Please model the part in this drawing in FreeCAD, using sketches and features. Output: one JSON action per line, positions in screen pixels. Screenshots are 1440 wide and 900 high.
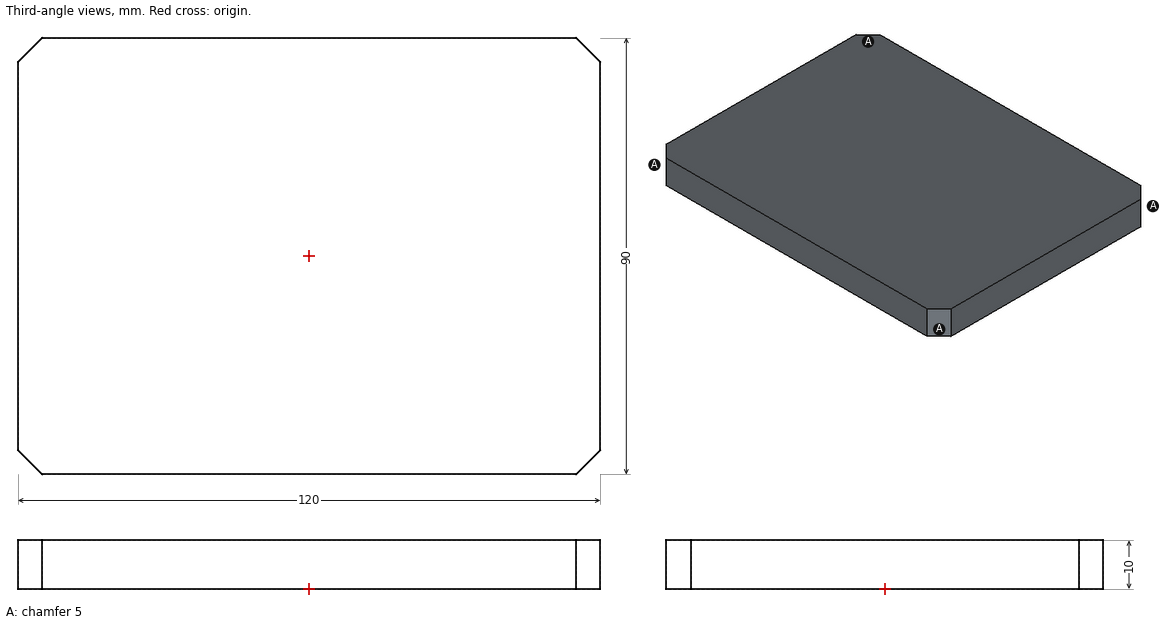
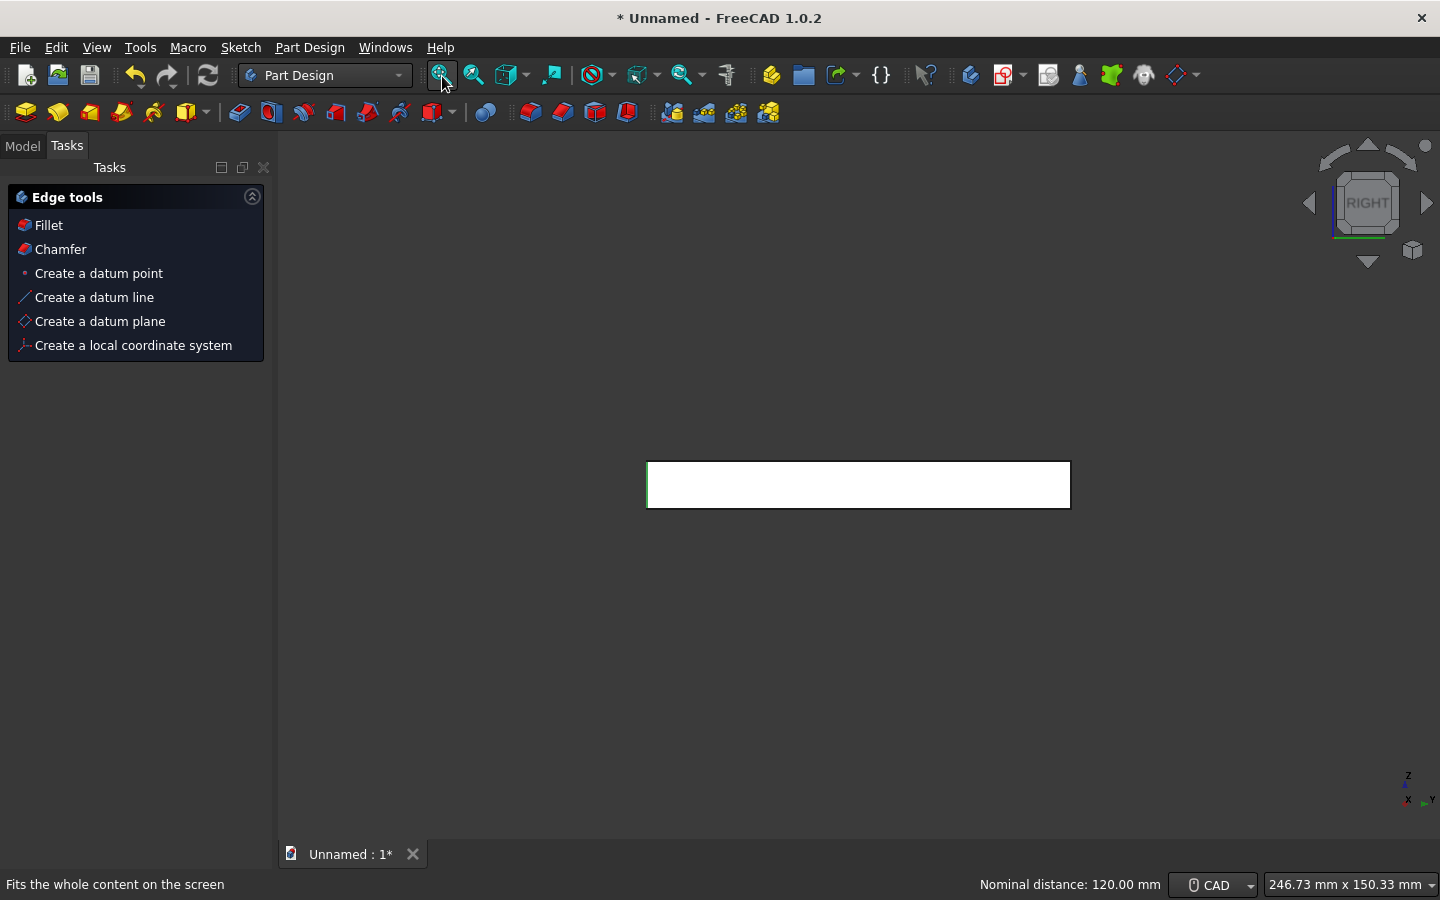
{"action": "left_click", "coordinate": [1071, 484], "text": "ctrl"}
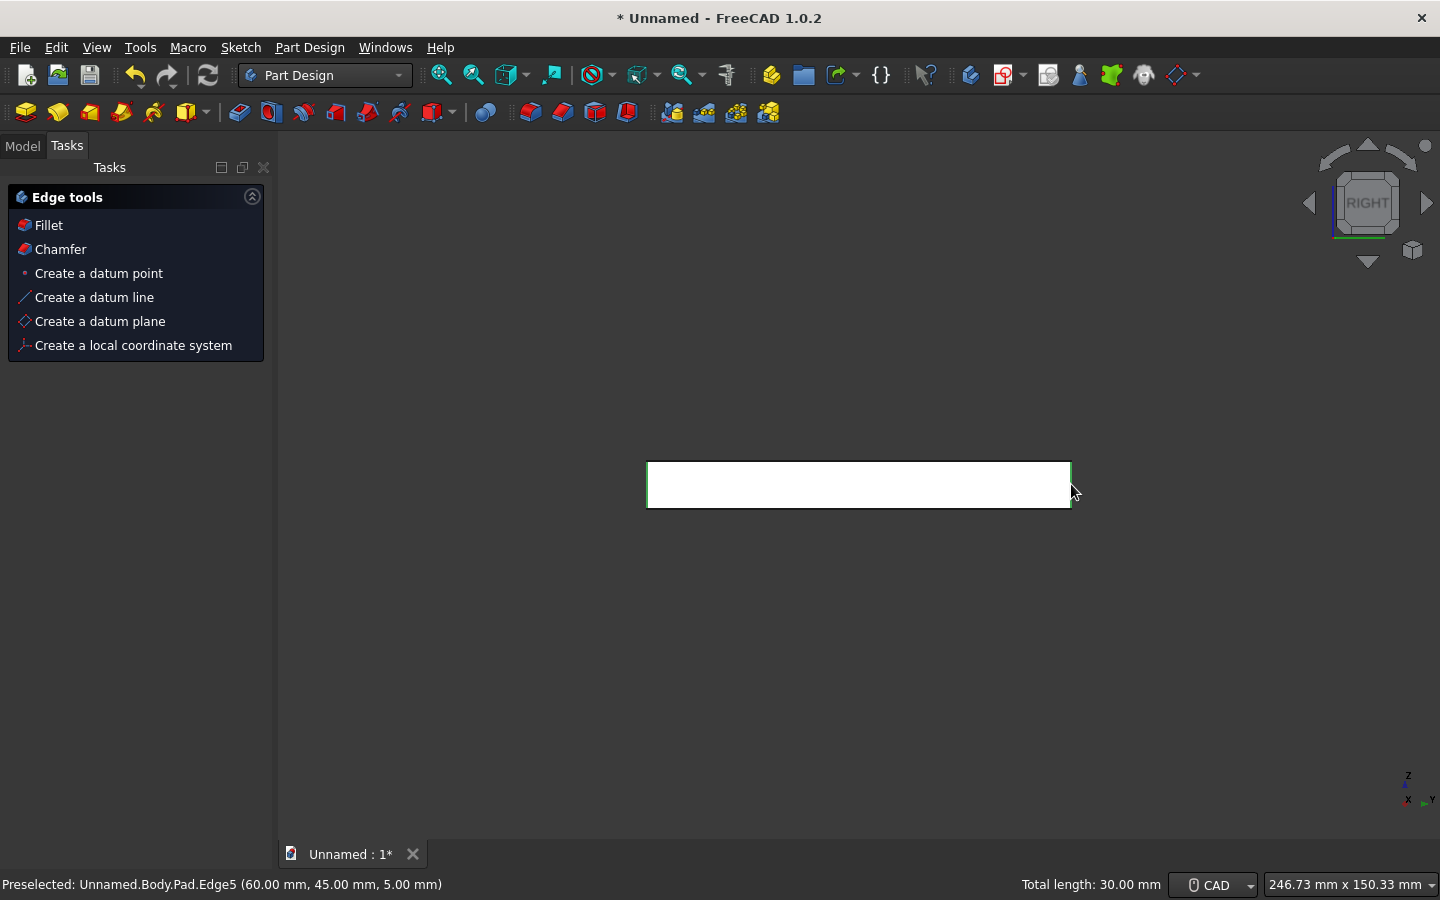
{"action": "key", "text": "5"}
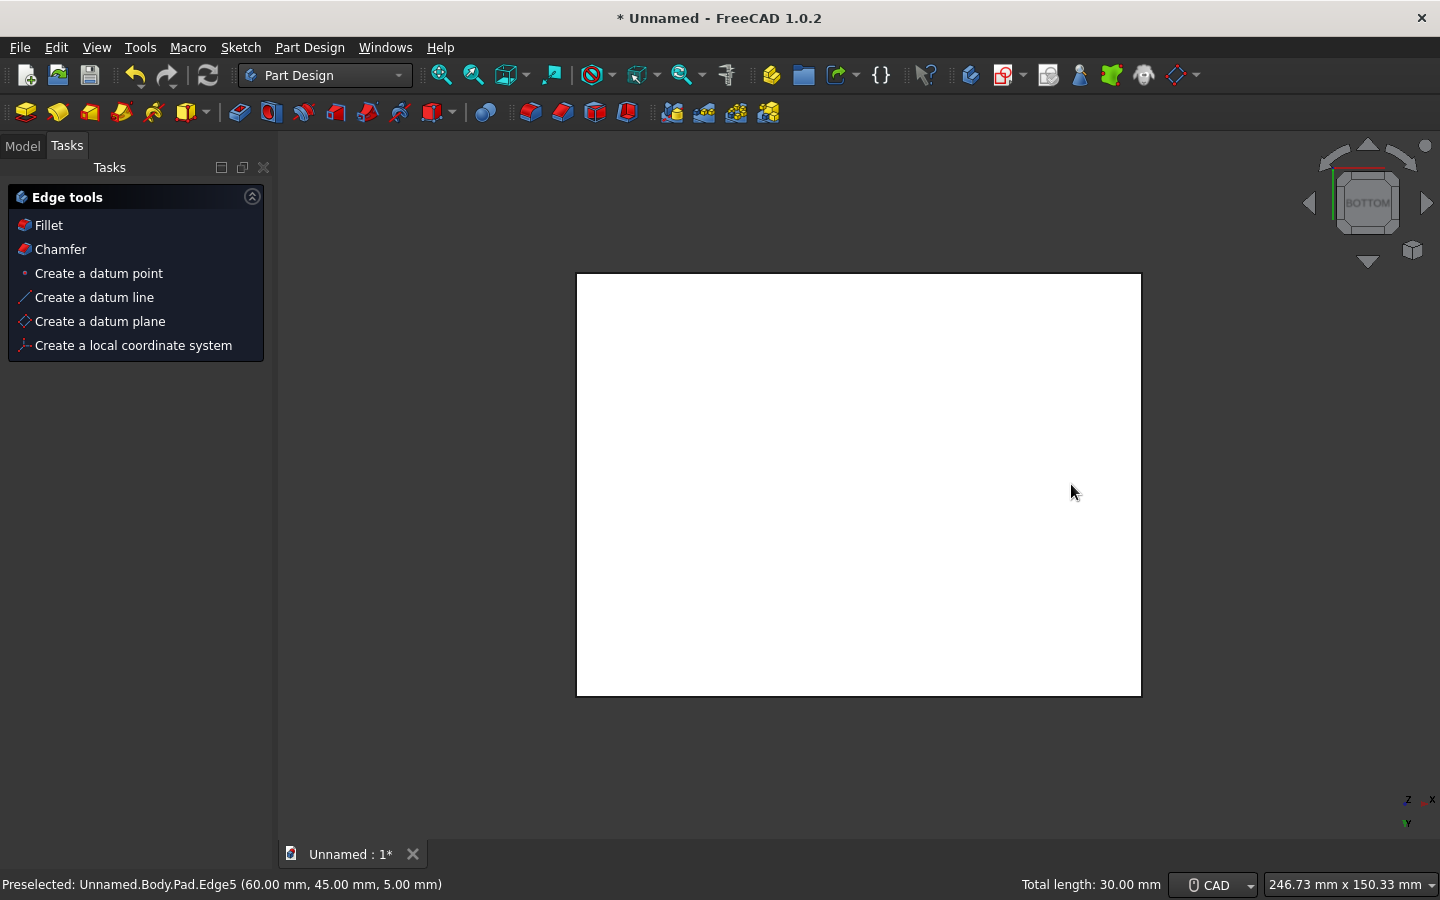
{"action": "key", "text": "4"}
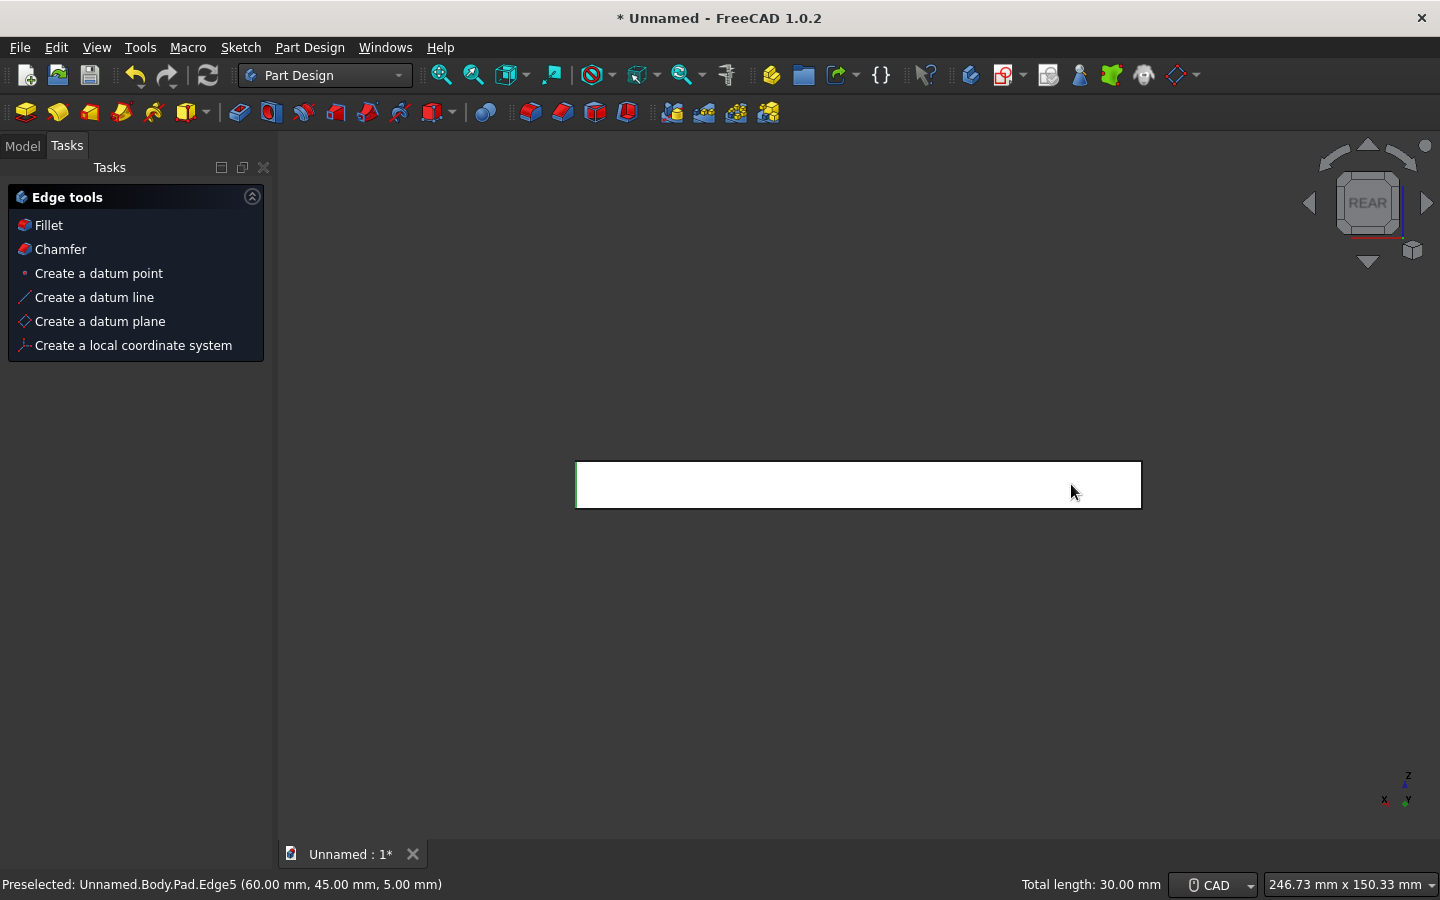
{"action": "left_click", "coordinate": [1142, 484], "text": "ctrl"}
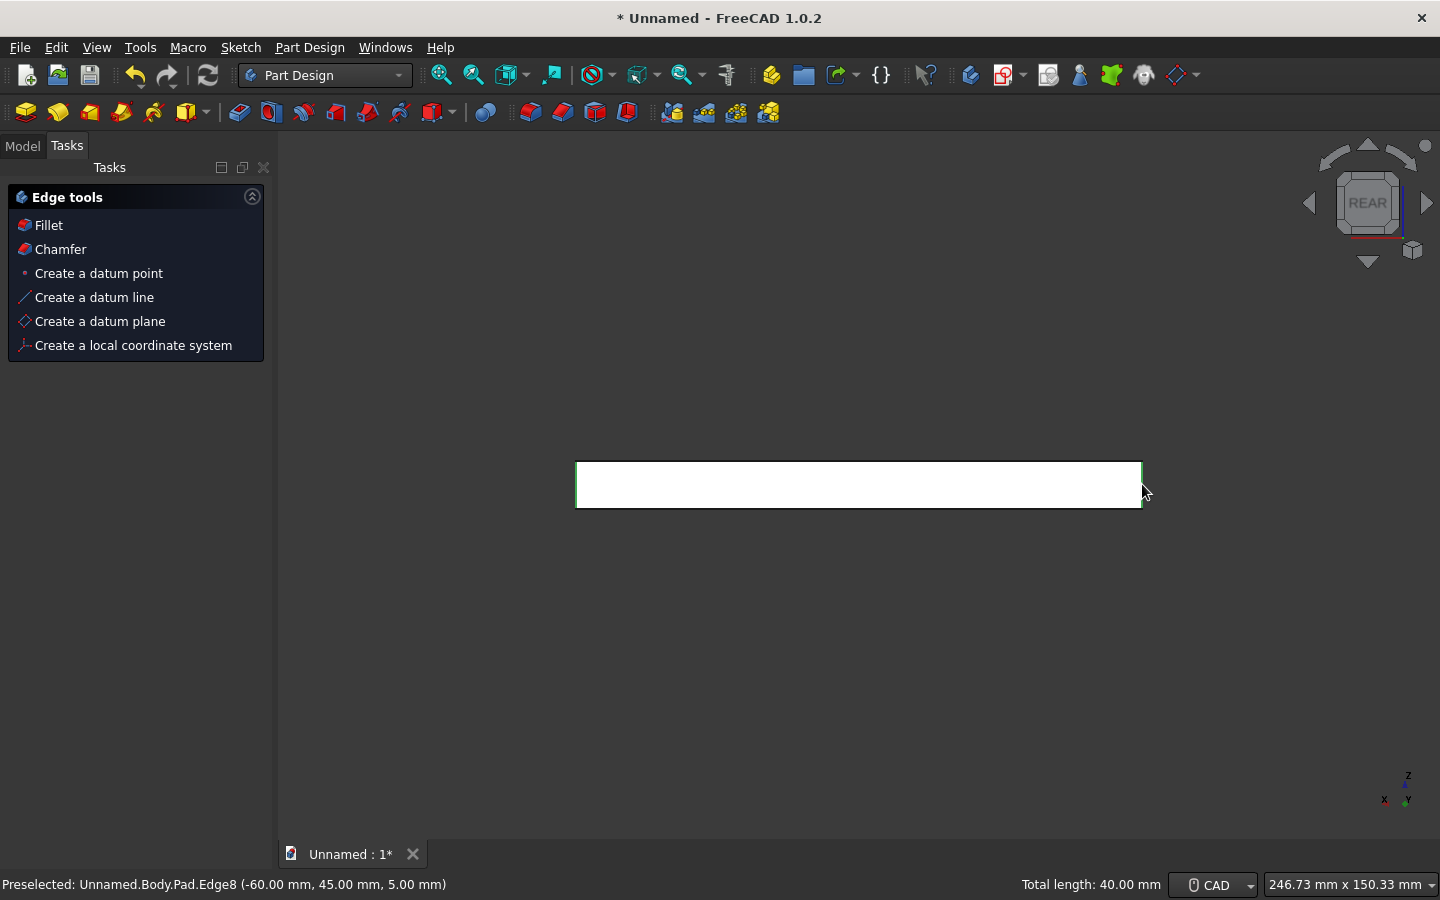
{"action": "left_click", "coordinate": [564, 112]}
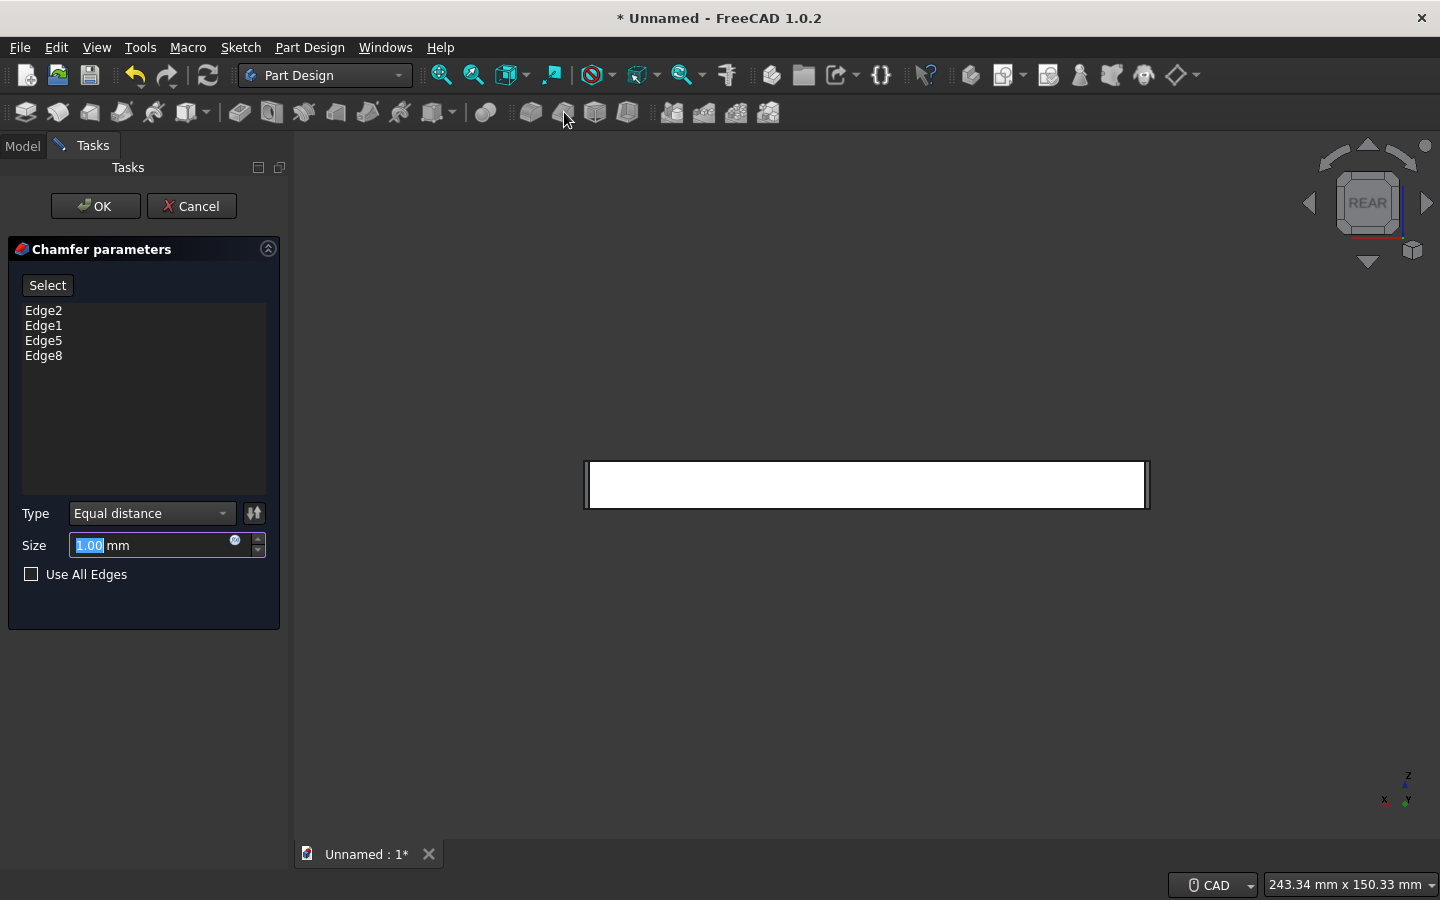
{"action": "type", "text": "5"}
{"action": "key", "text": "Tab"}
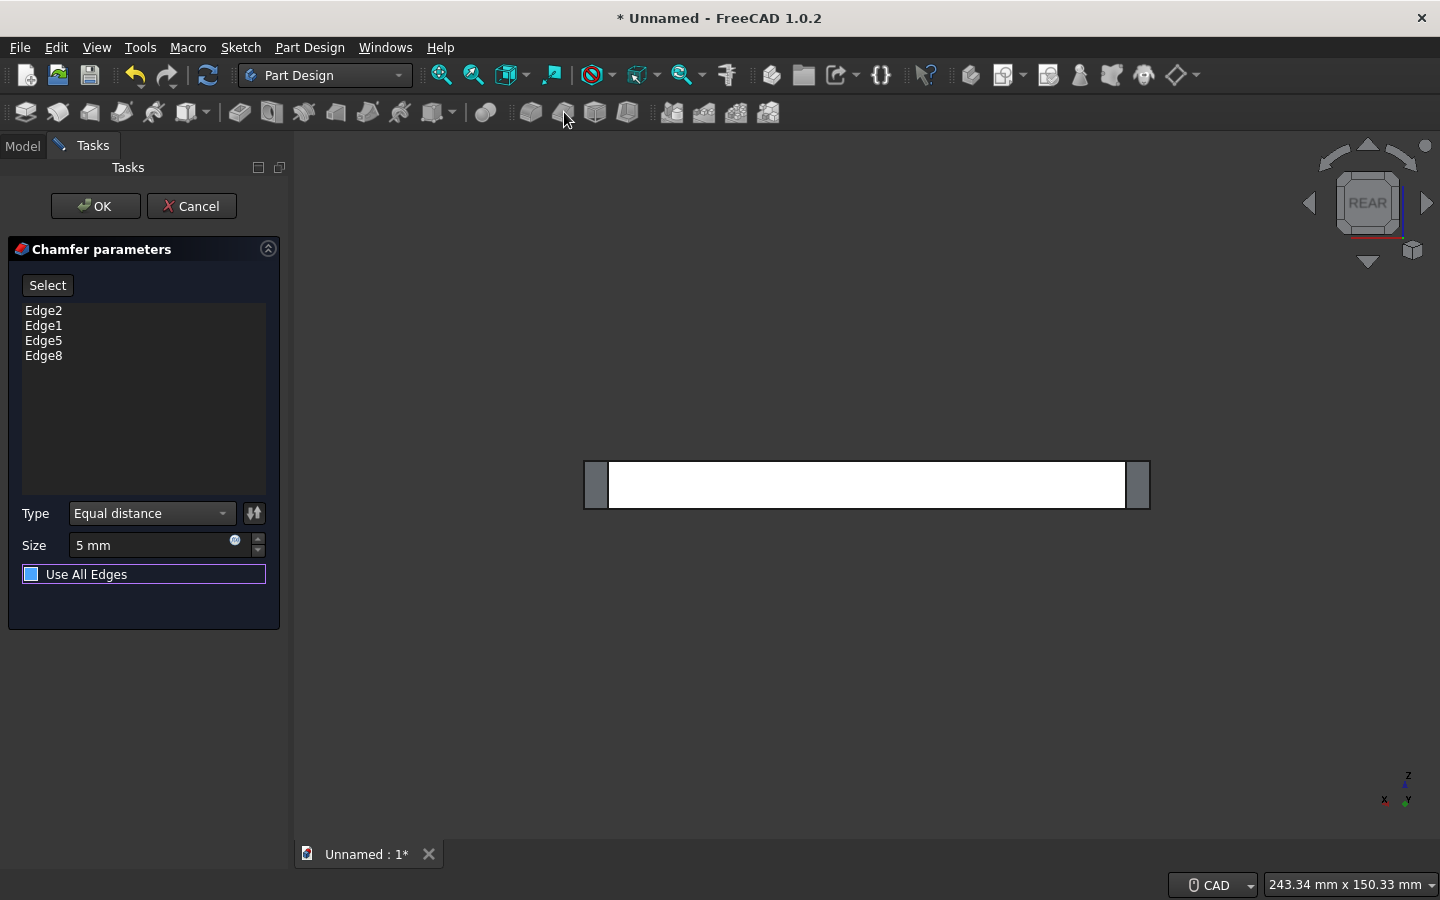
{"action": "left_click", "coordinate": [96, 206]}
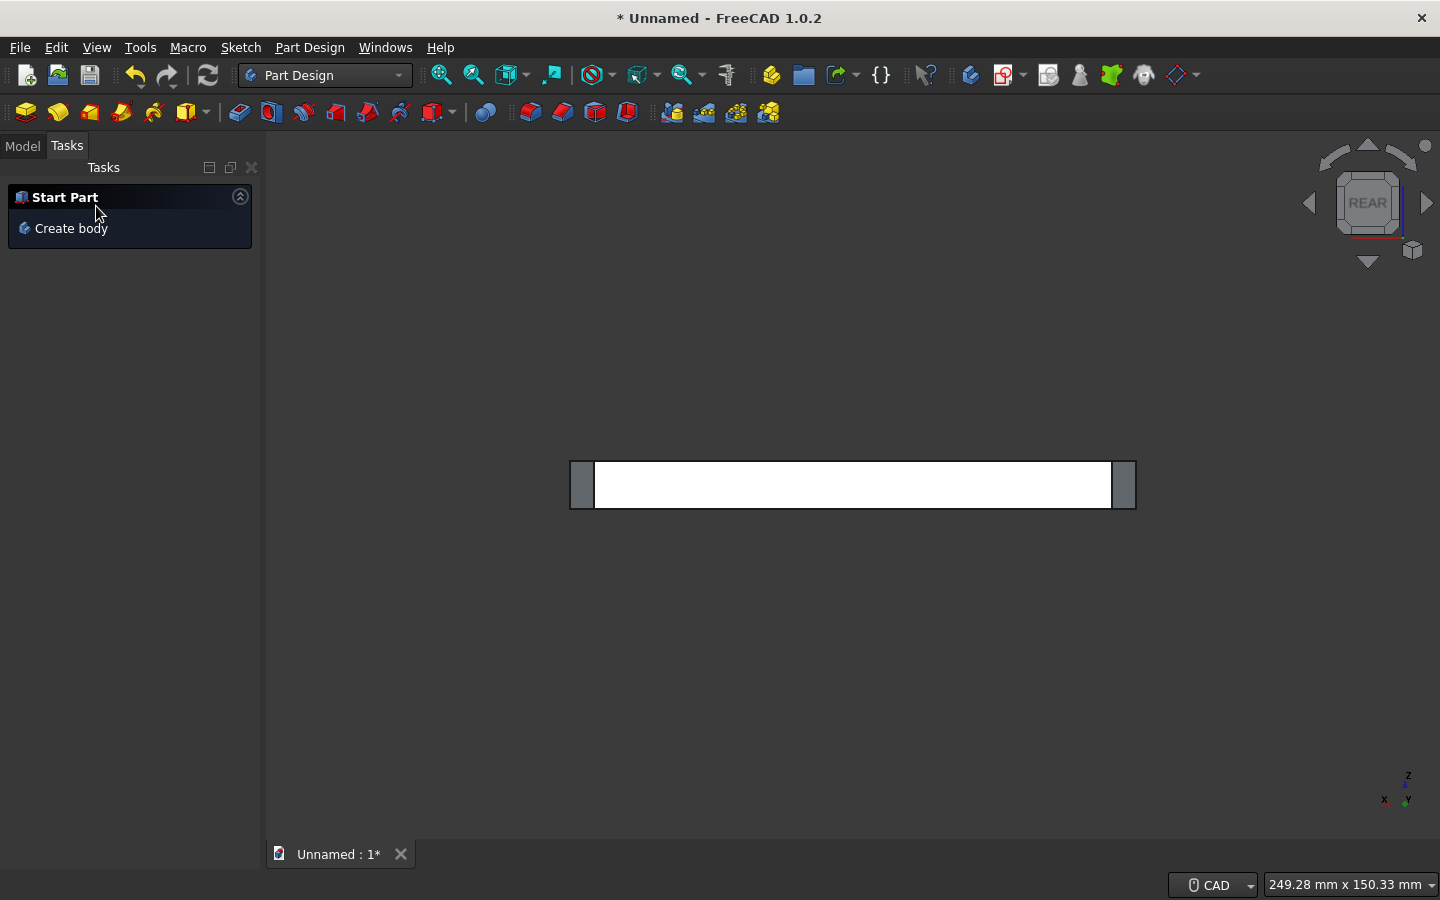
{"action": "key", "text": "0"}